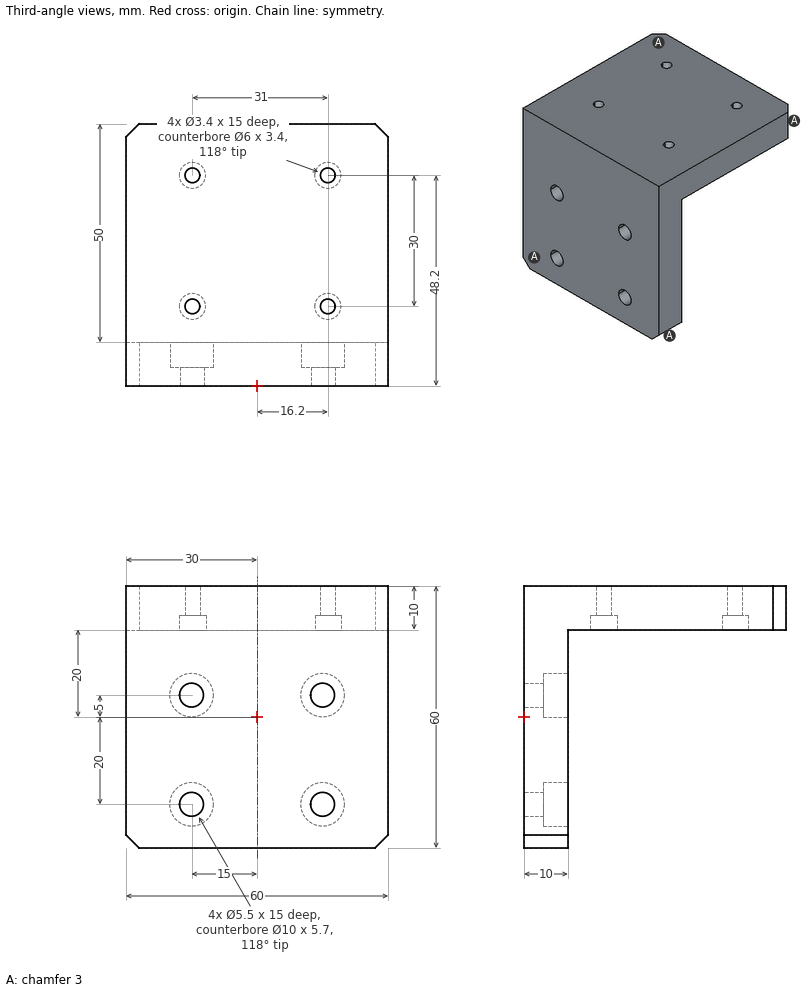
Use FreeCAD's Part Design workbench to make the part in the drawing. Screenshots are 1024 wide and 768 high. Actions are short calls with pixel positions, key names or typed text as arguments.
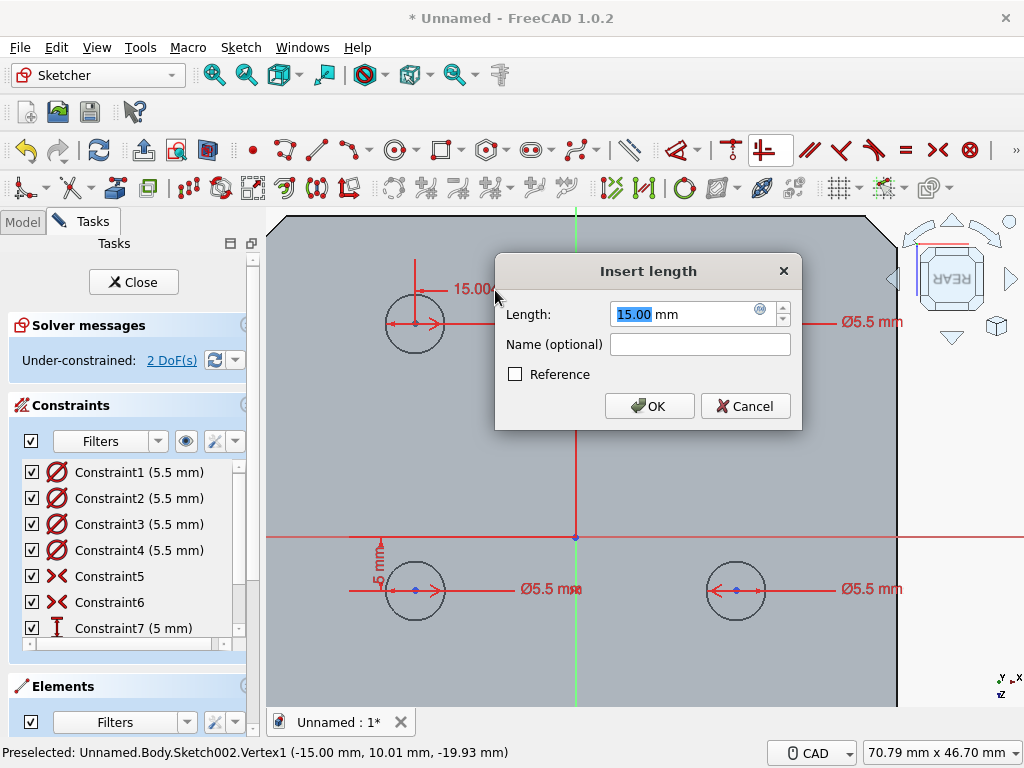
text(15)
key(Return)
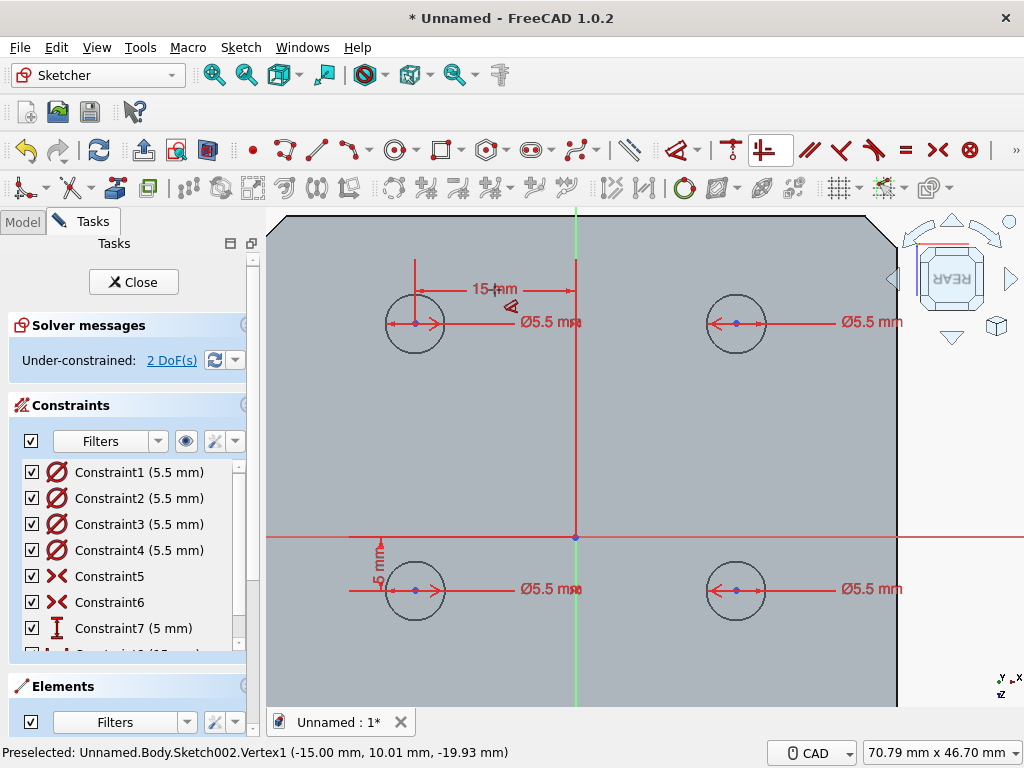
click(415, 324)
click(381, 431)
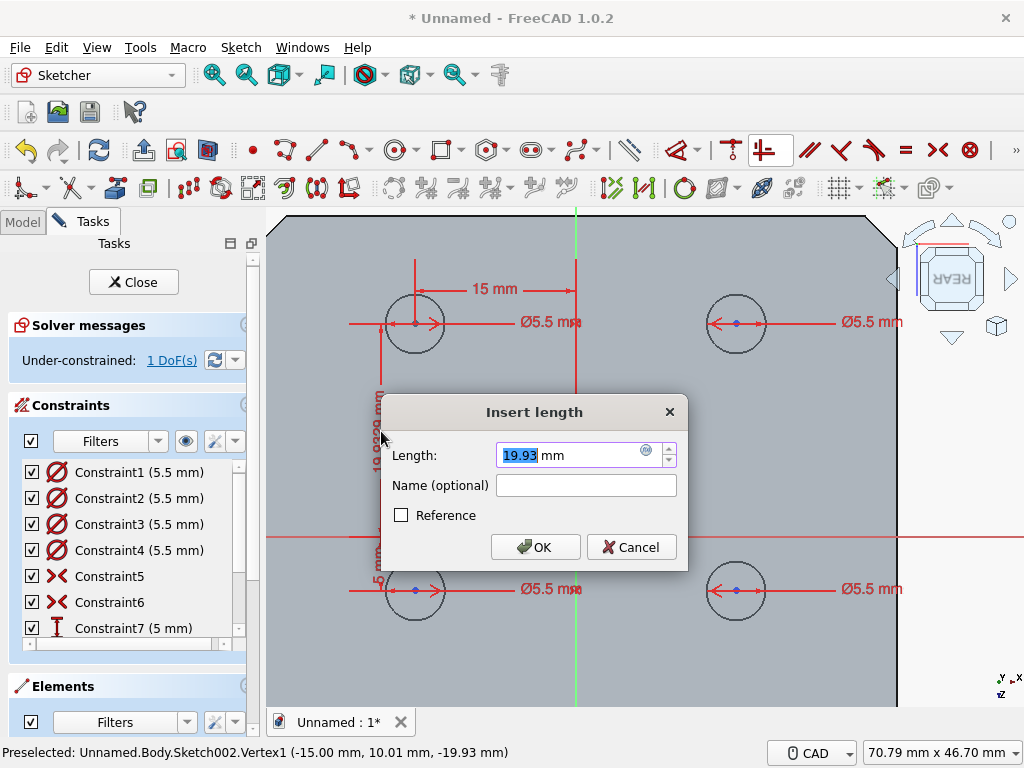
text(20)
key(Return)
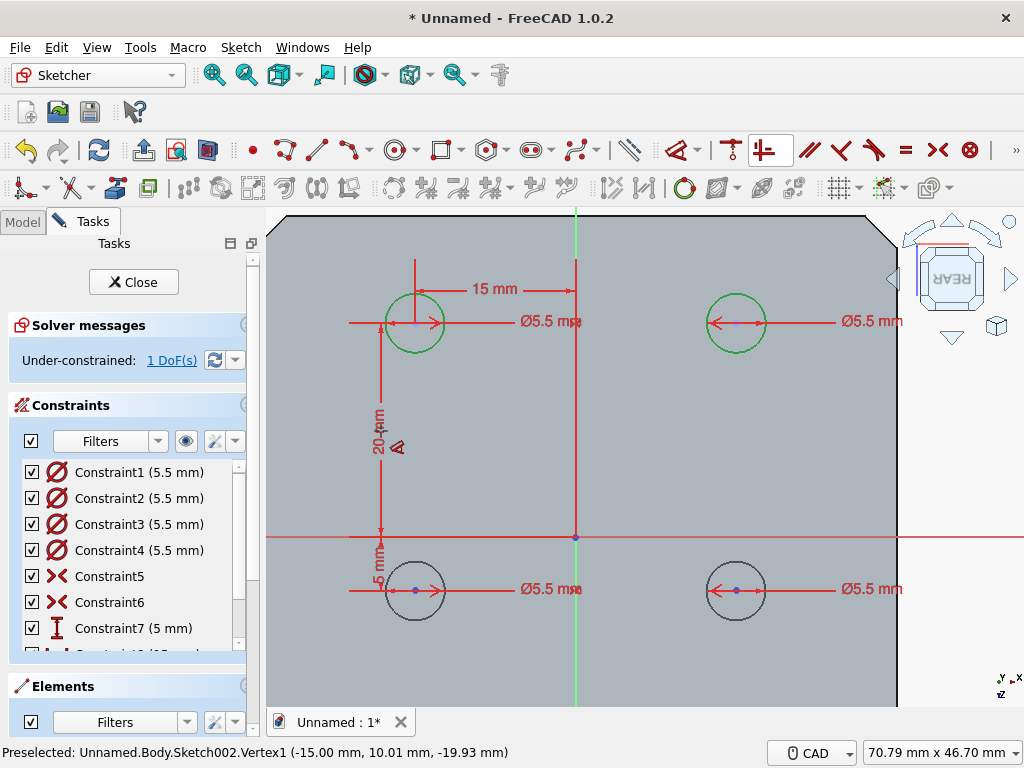
click(415, 591)
click(495, 625)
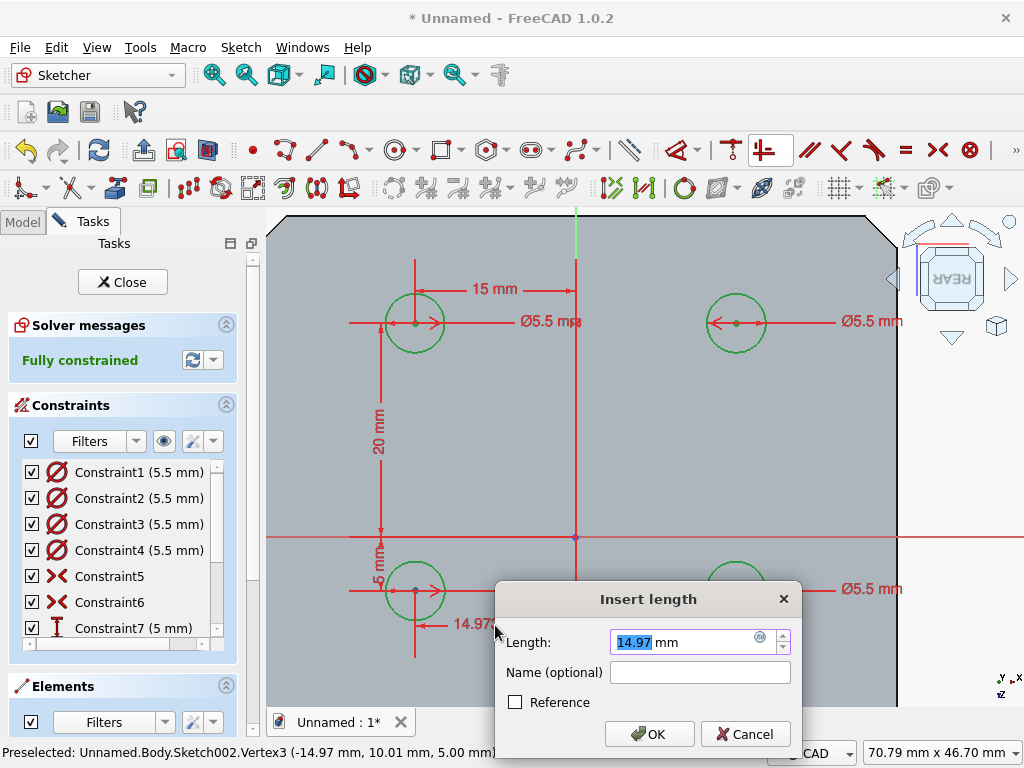
text(15)
key(Return)
key(Escape)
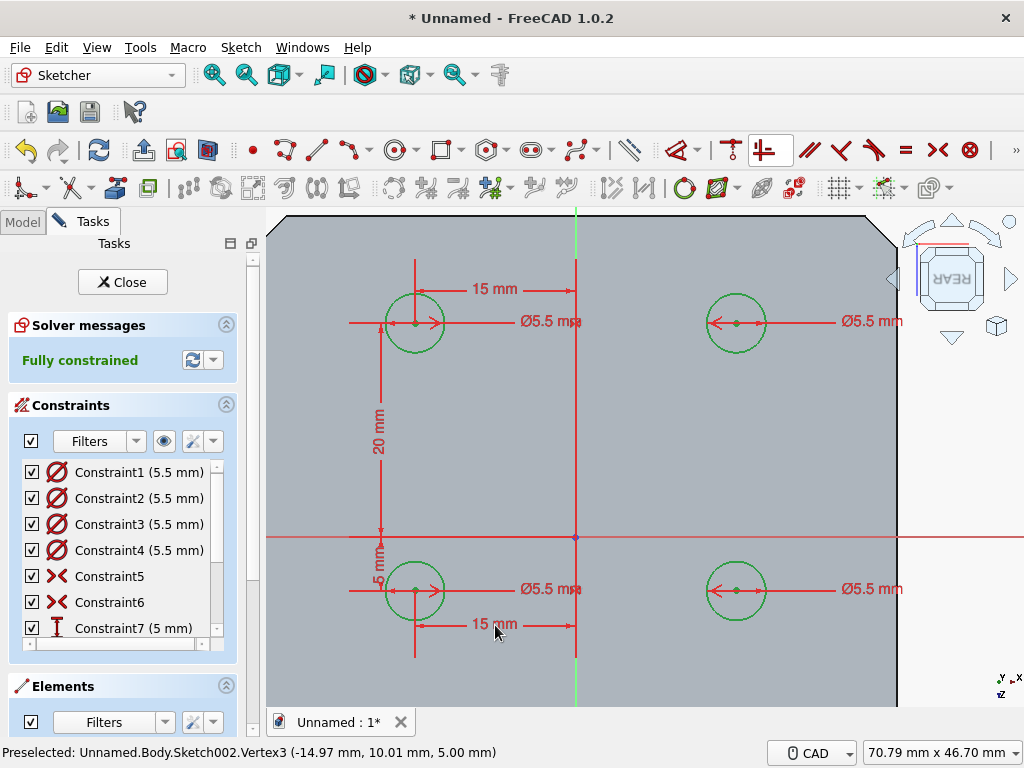
click(123, 282)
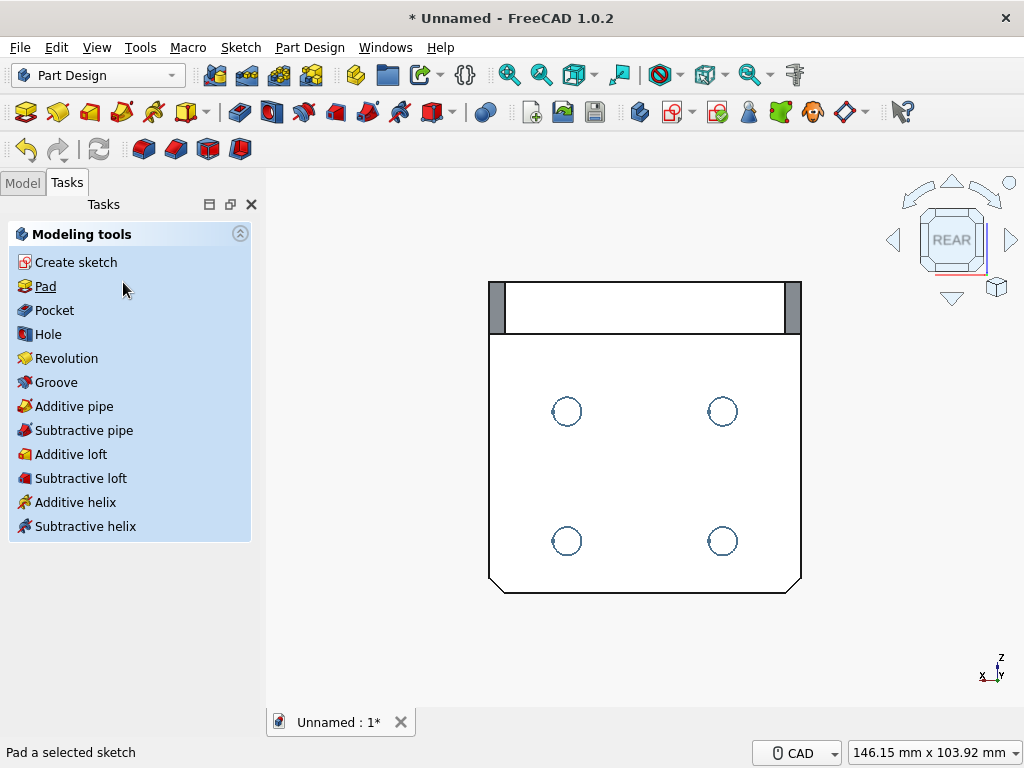
click(272, 112)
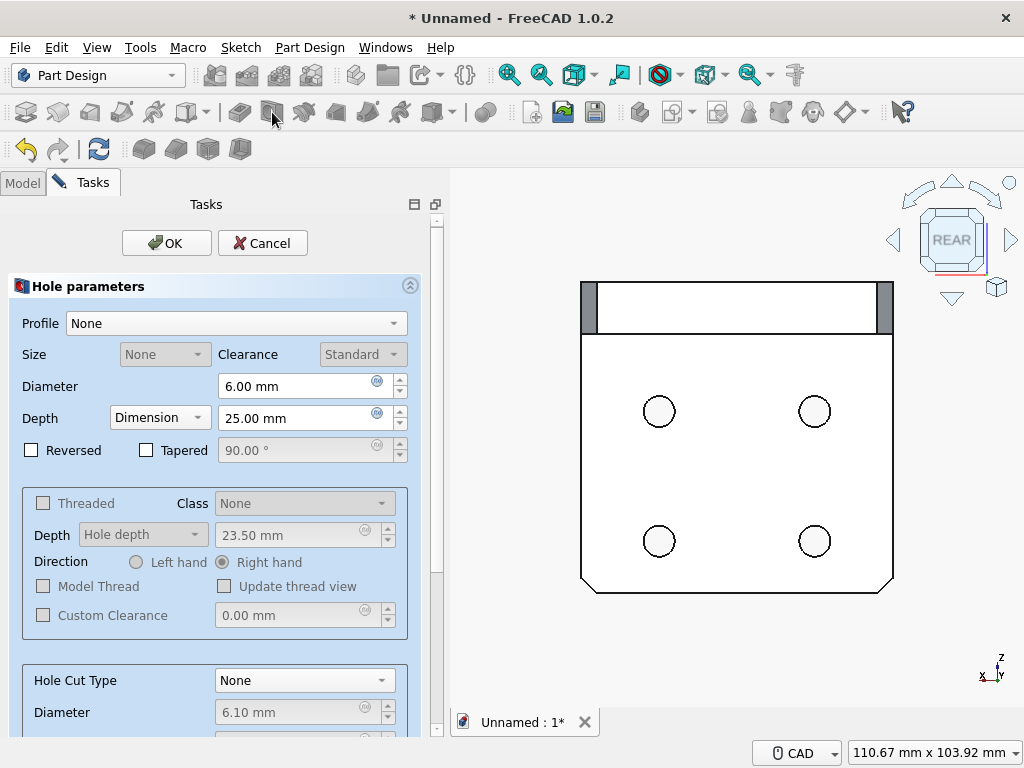
triple_click(305, 386)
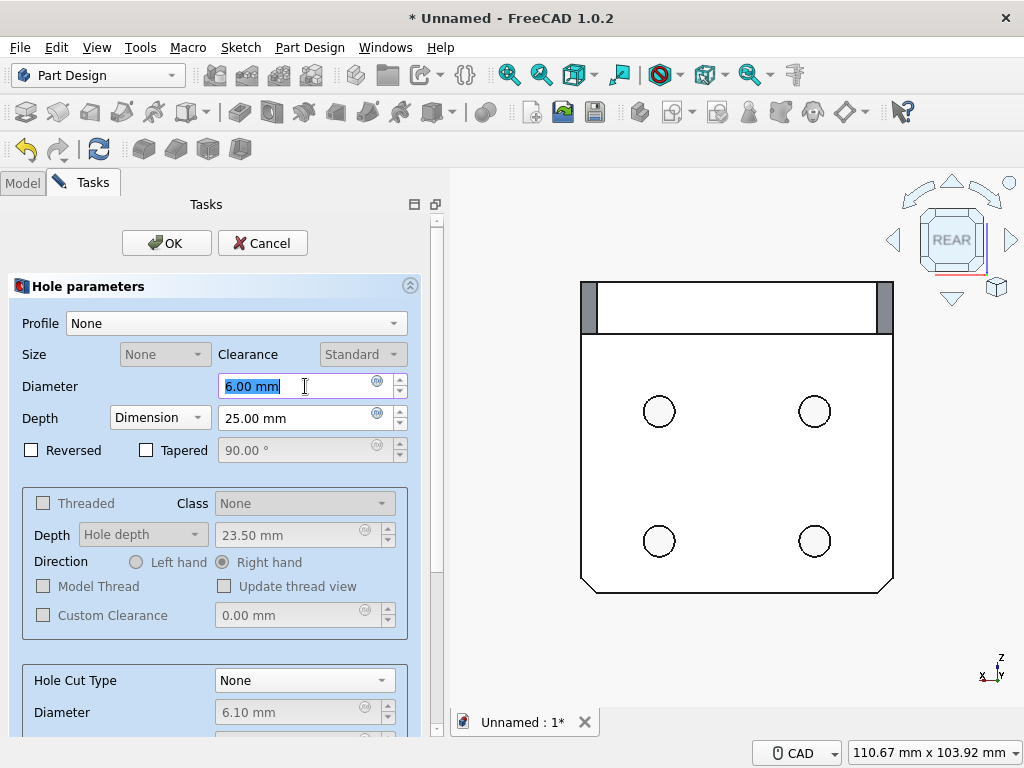
text(5.5)
key(Tab)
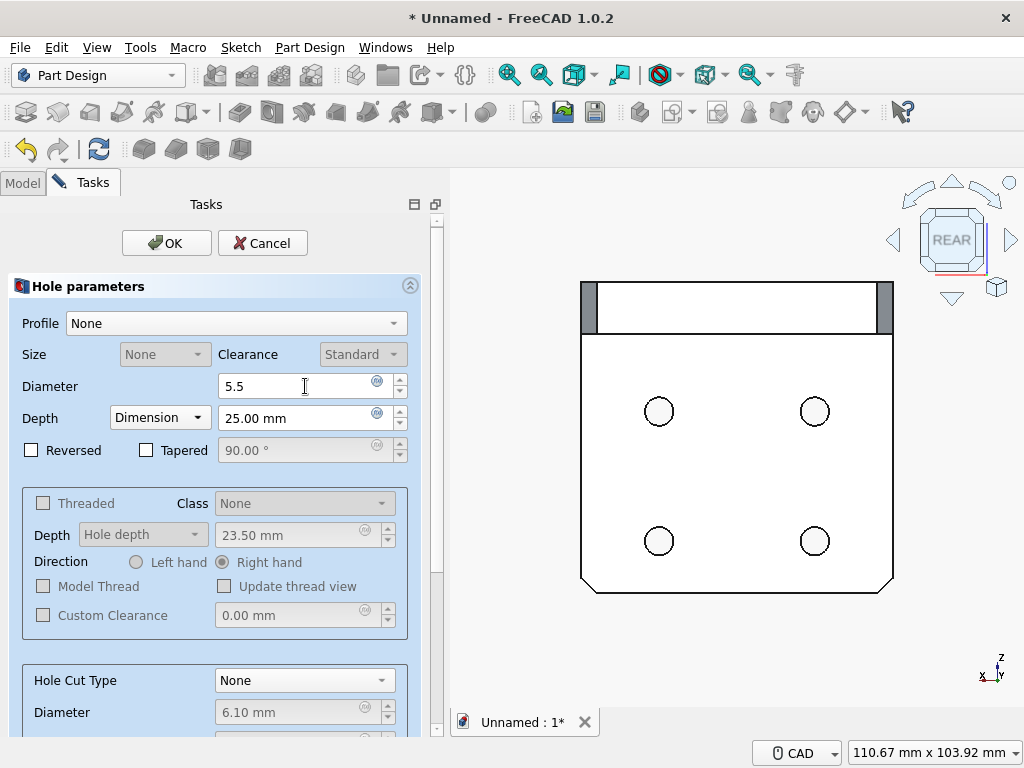
triple_click(305, 418)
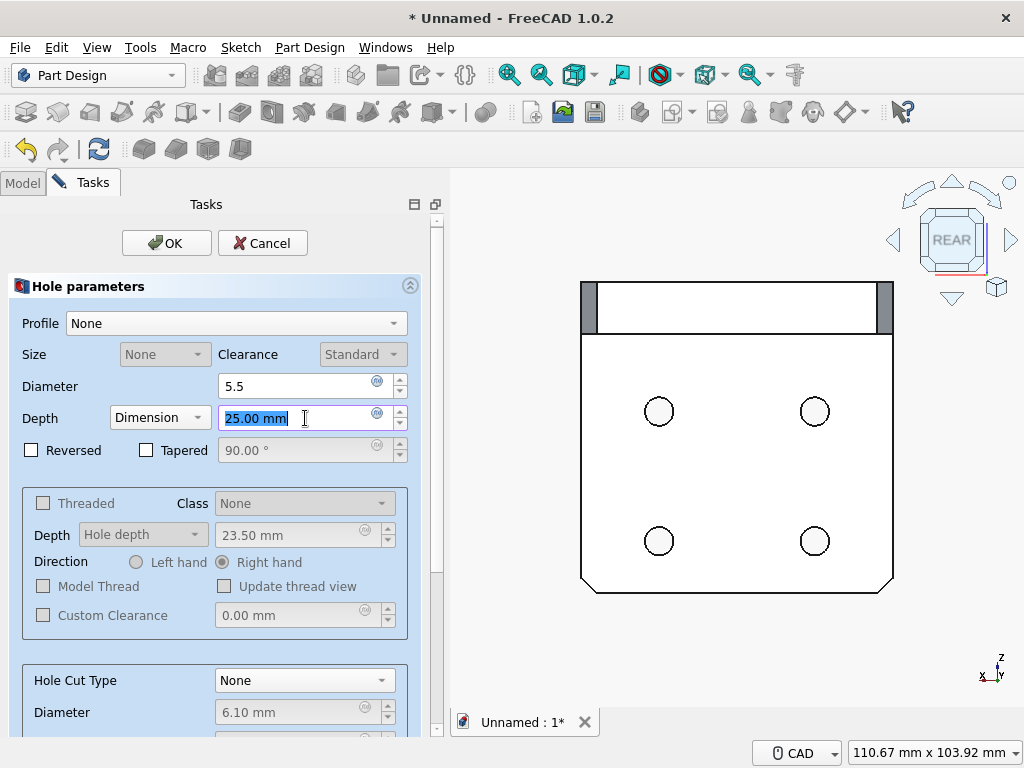
text(15)
key(Tab)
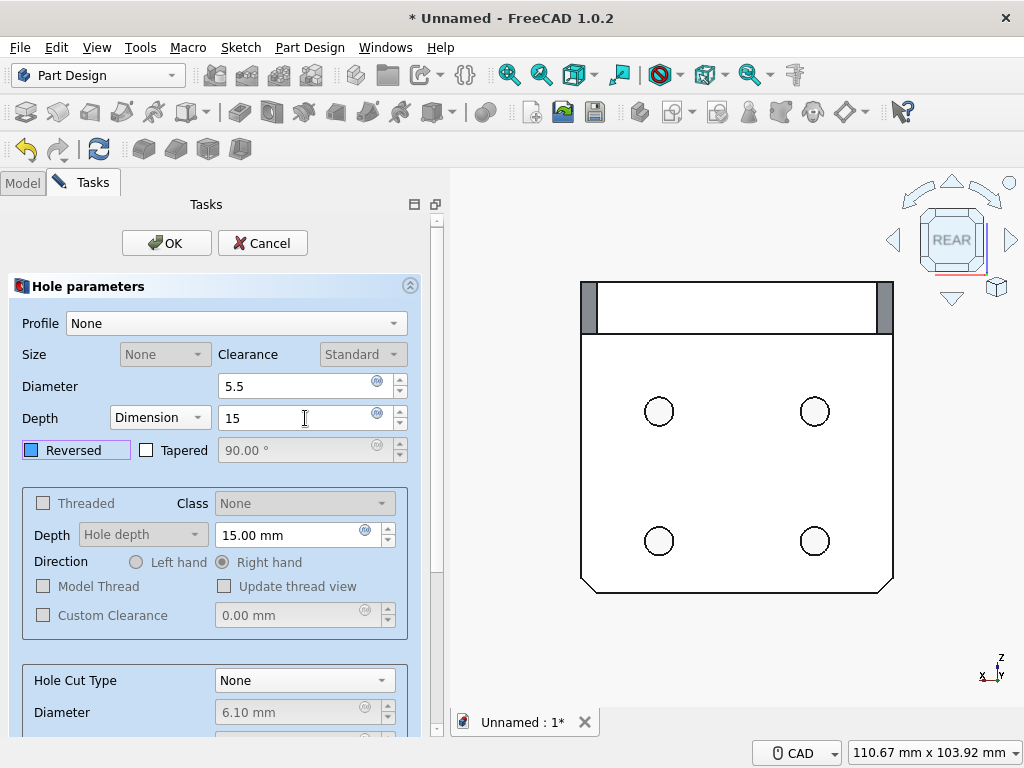
click(306, 680)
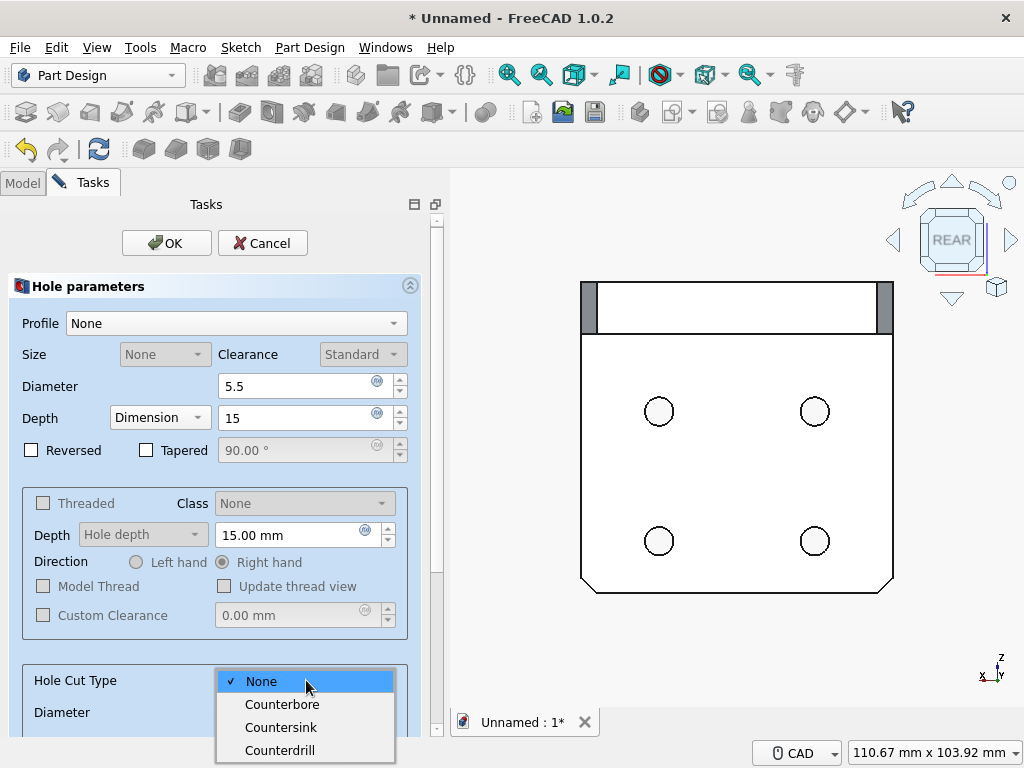
click(304, 704)